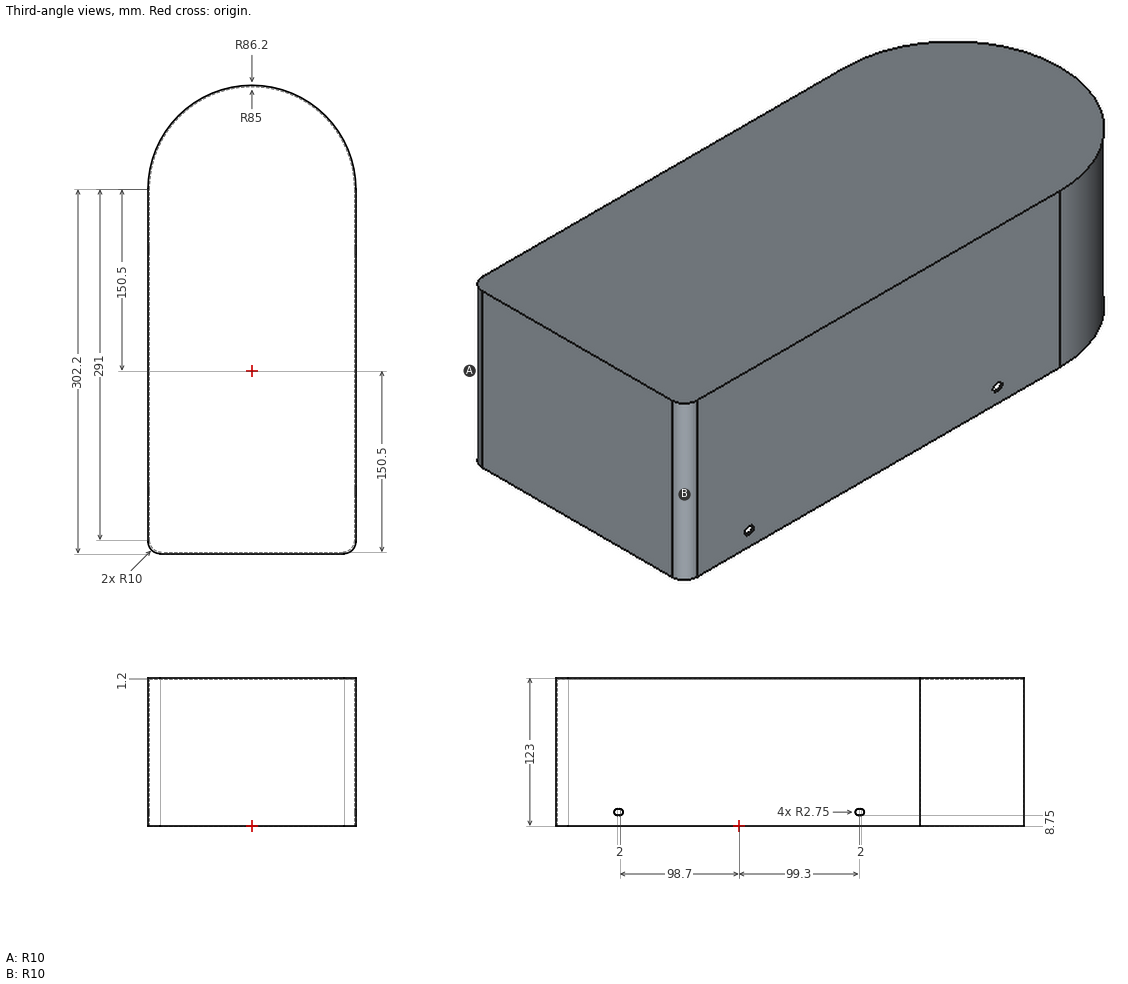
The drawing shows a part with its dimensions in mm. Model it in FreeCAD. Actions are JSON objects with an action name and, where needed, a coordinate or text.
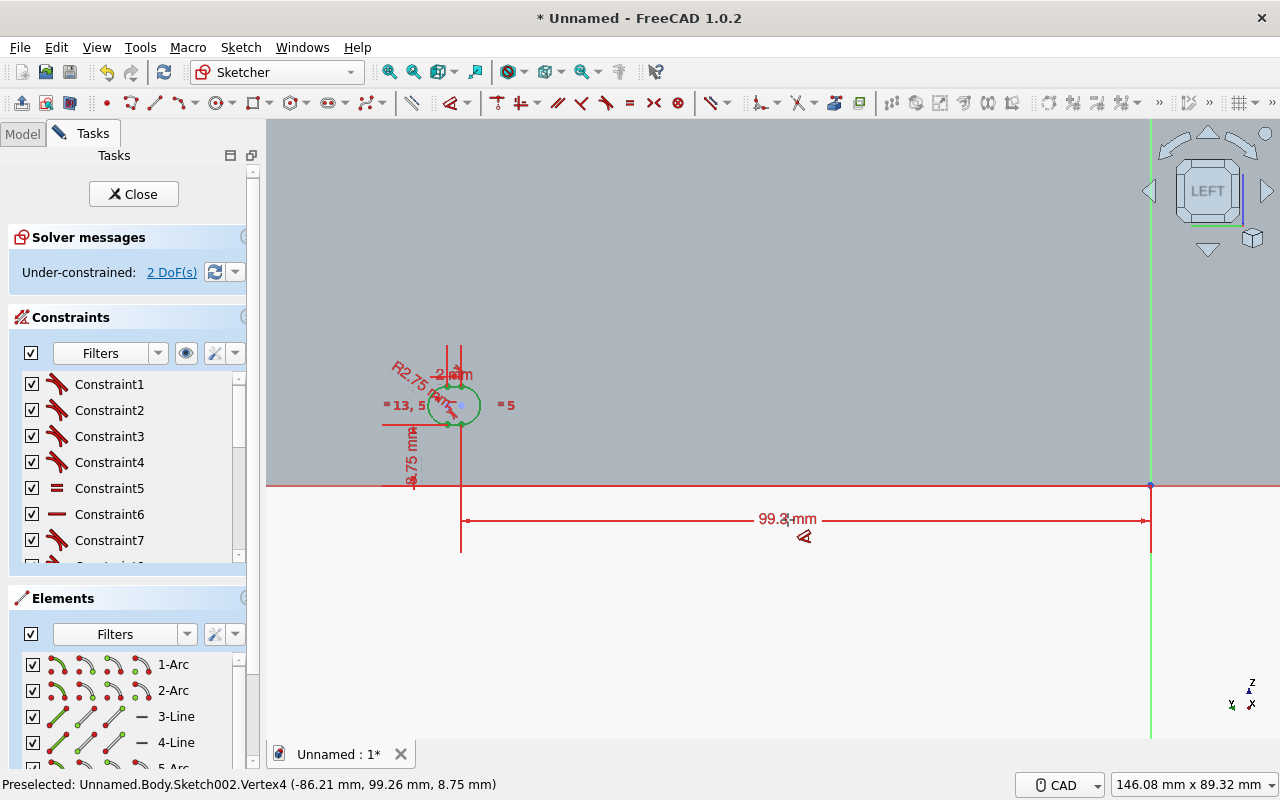
{"action": "scroll", "coordinate": [446, 425], "scroll_direction": "down", "scroll_amount": 5}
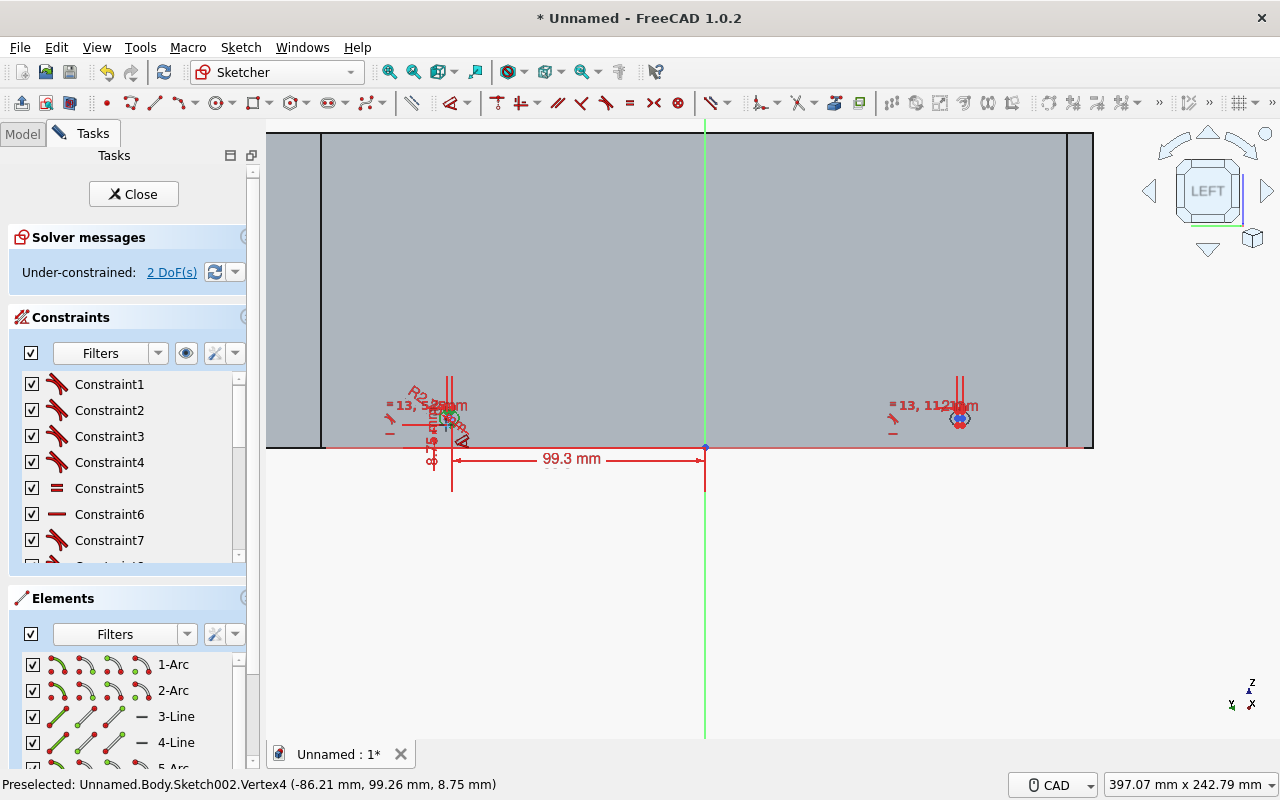
{"action": "scroll", "coordinate": [957, 412], "scroll_direction": "up", "scroll_amount": 5}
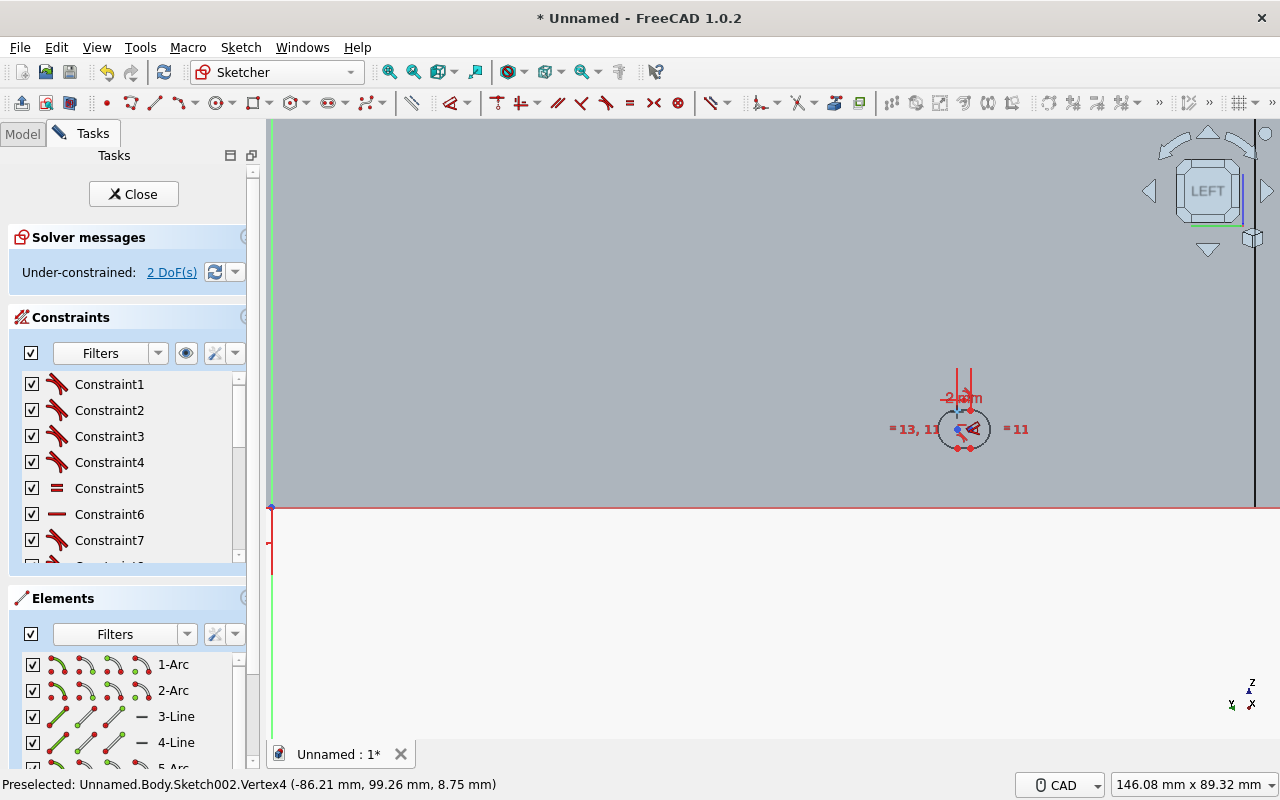
{"action": "left_click", "coordinate": [957, 410]}
{"action": "left_click", "coordinate": [626, 542]}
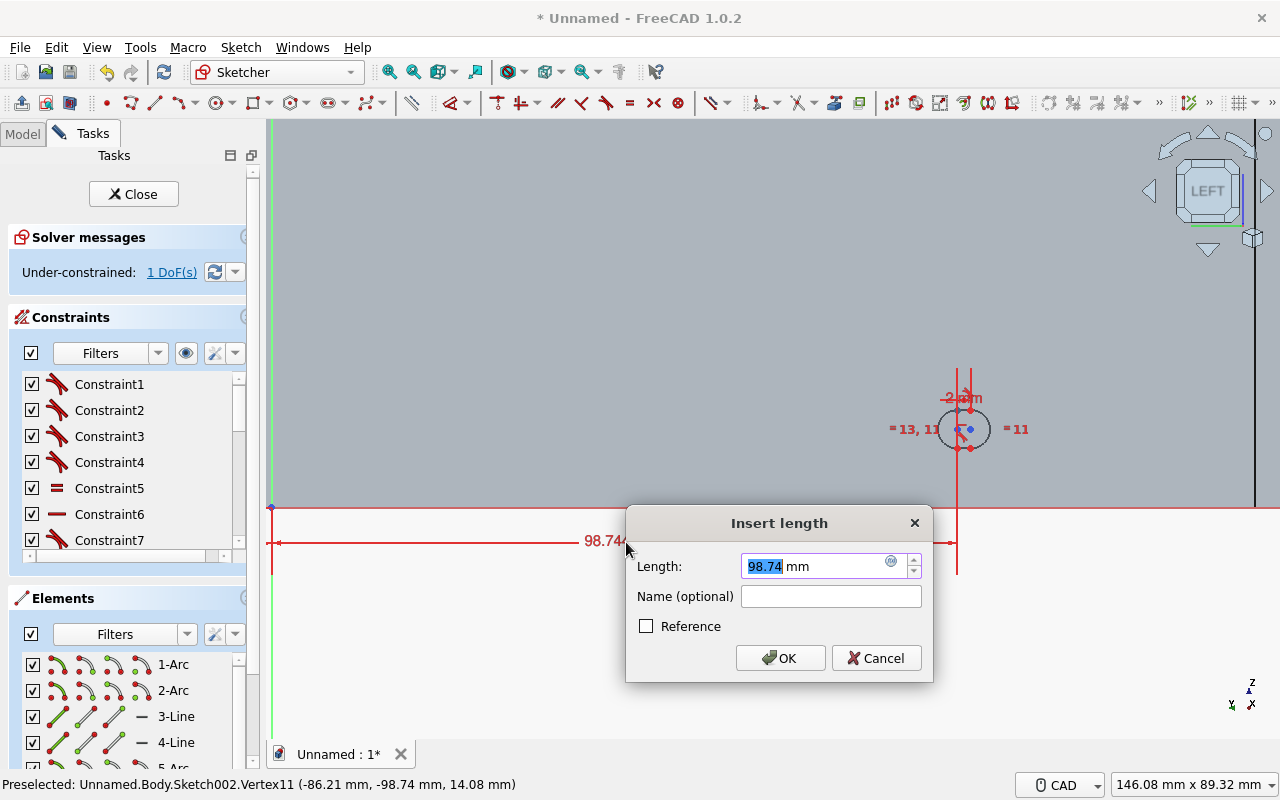
{"action": "type", "text": "98.7"}
{"action": "key", "text": "Return"}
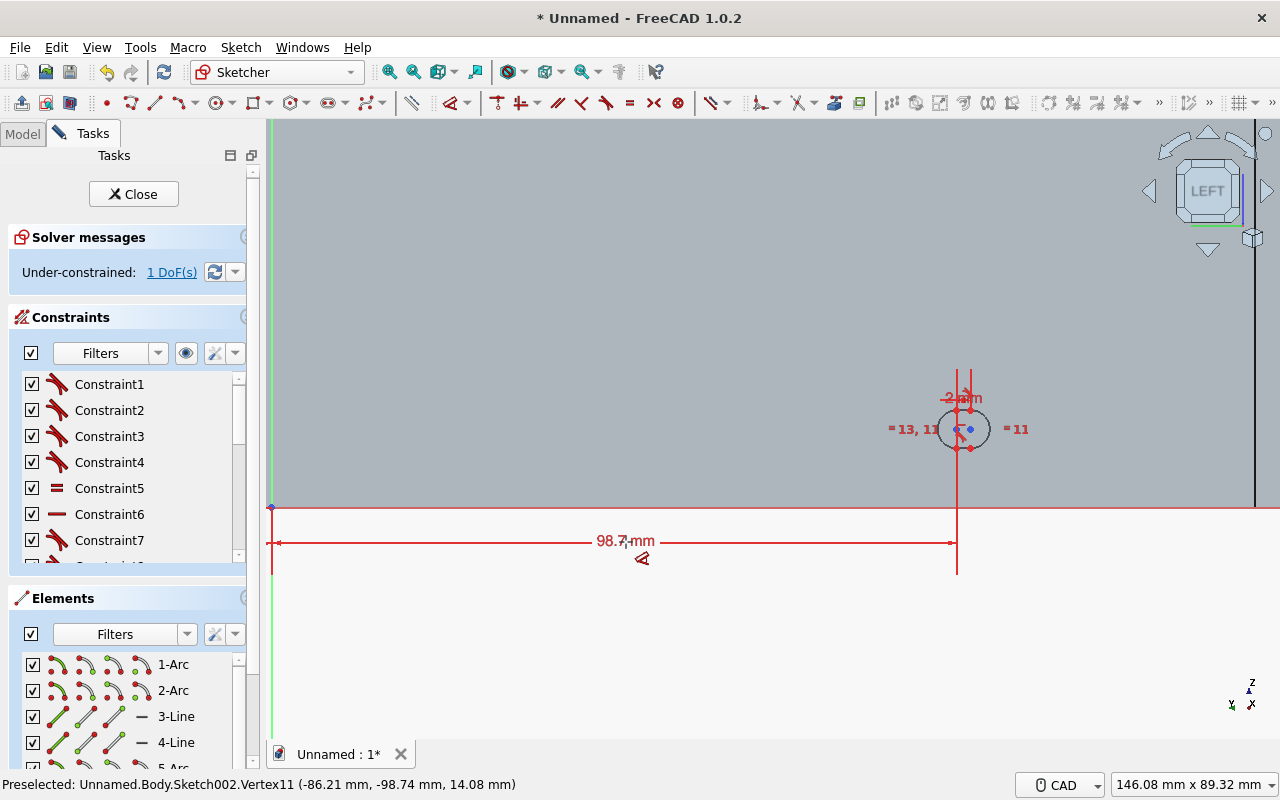
{"action": "left_click", "coordinate": [957, 448]}
{"action": "left_click", "coordinate": [991, 478]}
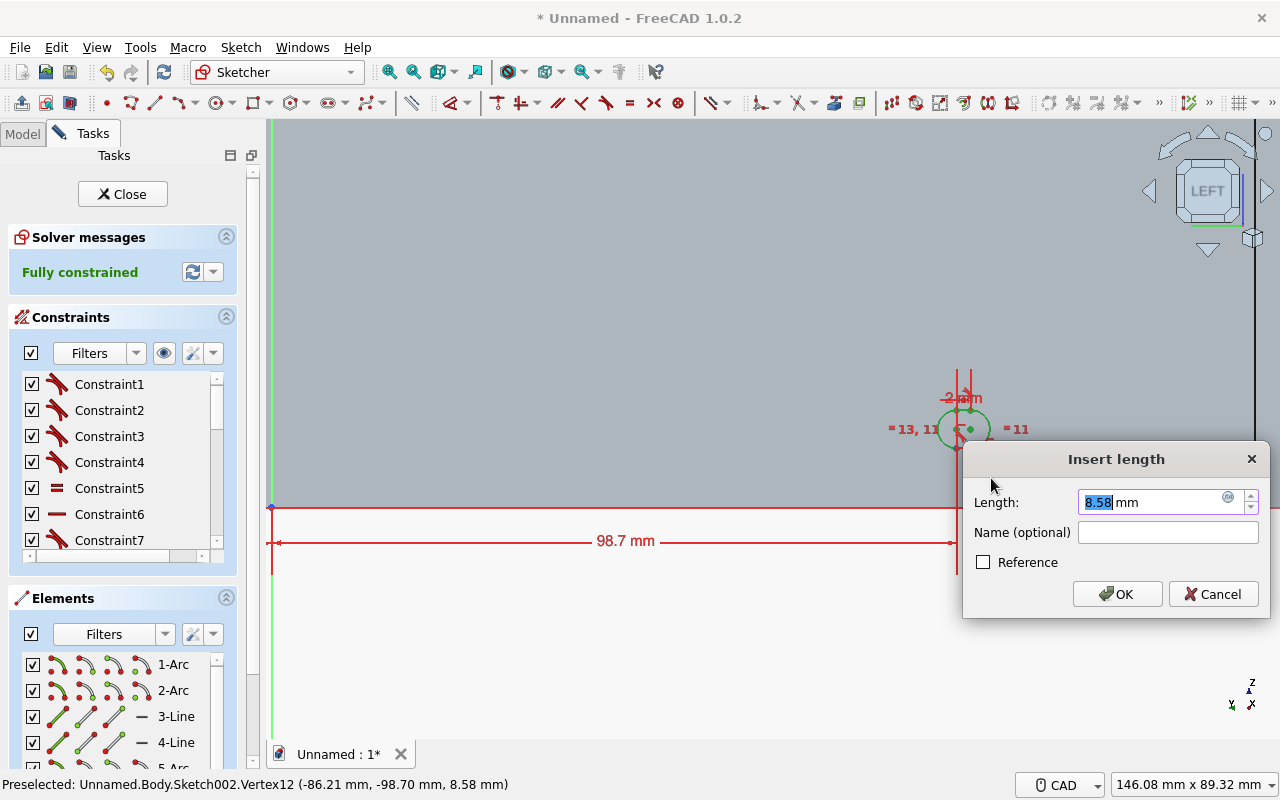
{"action": "type", "text": "8.75"}
{"action": "key", "text": "Return"}
{"action": "key", "text": "Escape"}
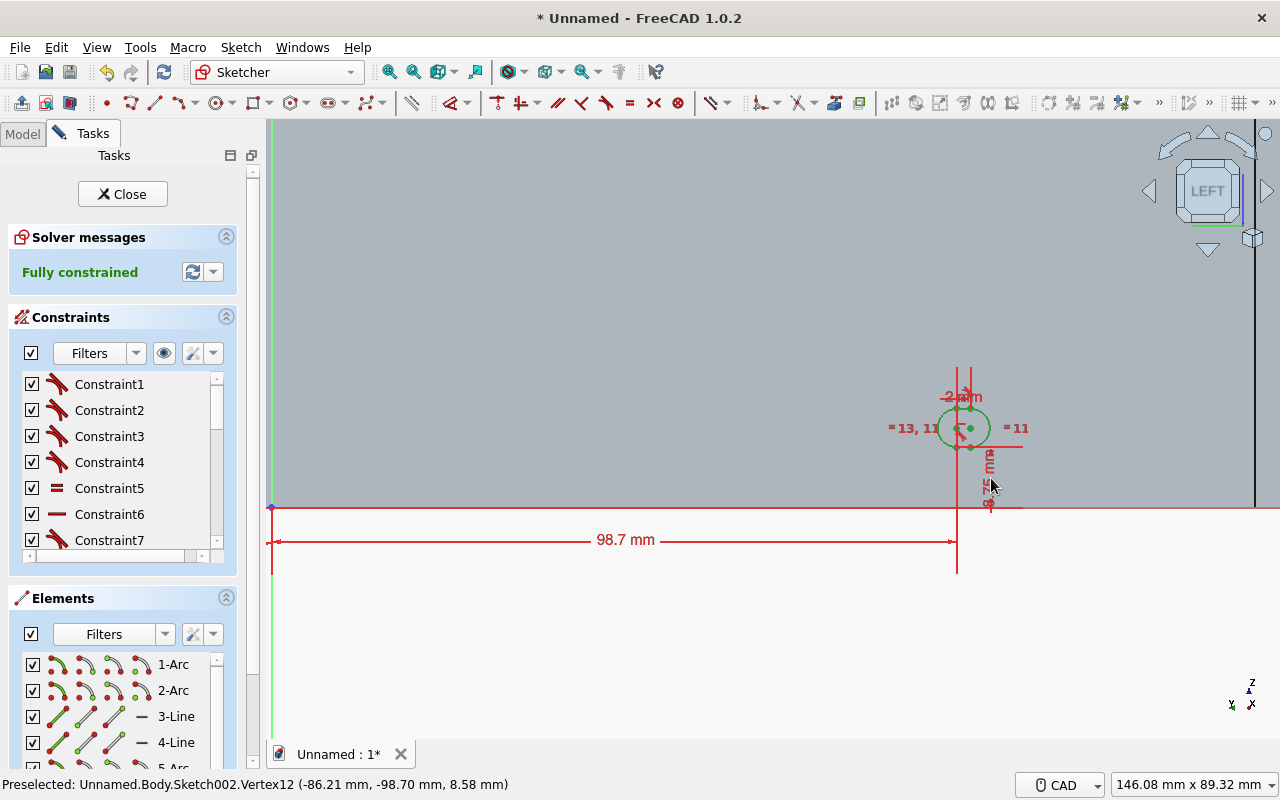
{"action": "left_click", "coordinate": [123, 194]}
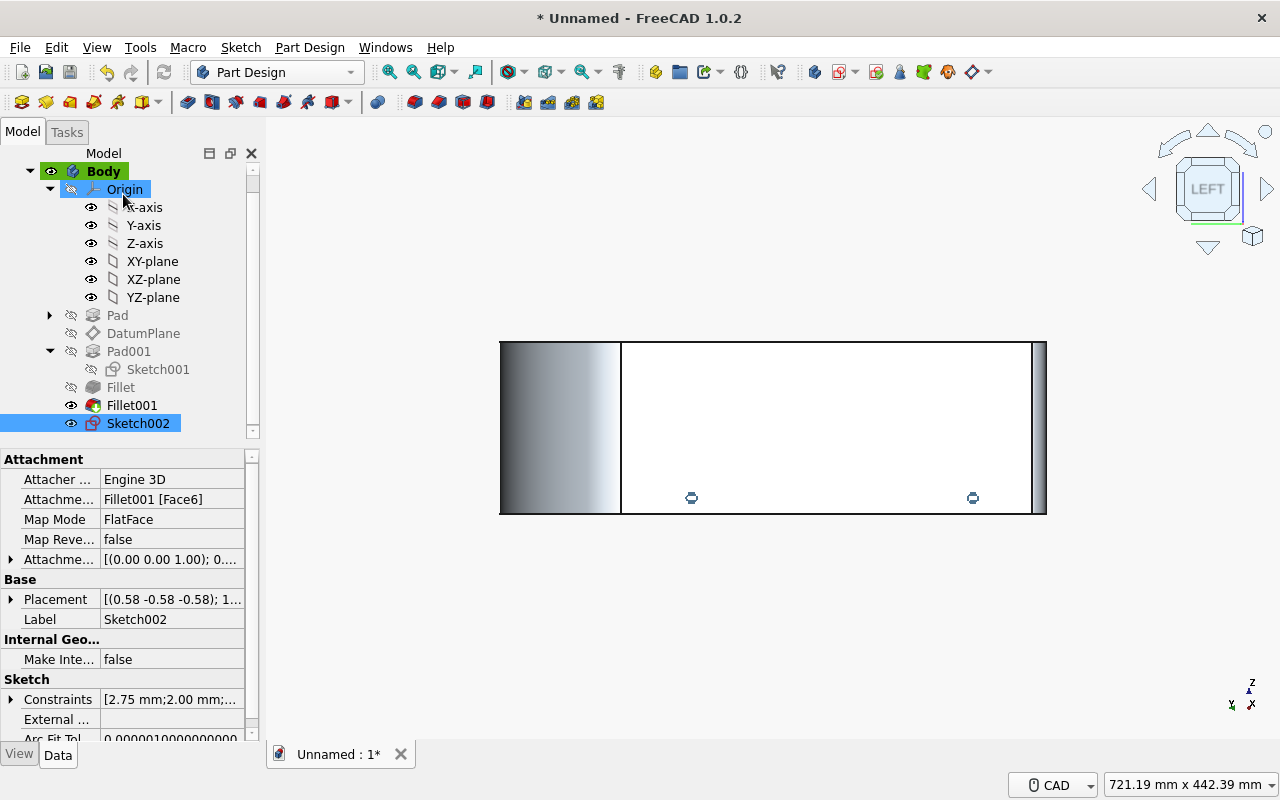
{"action": "left_click", "coordinate": [188, 102]}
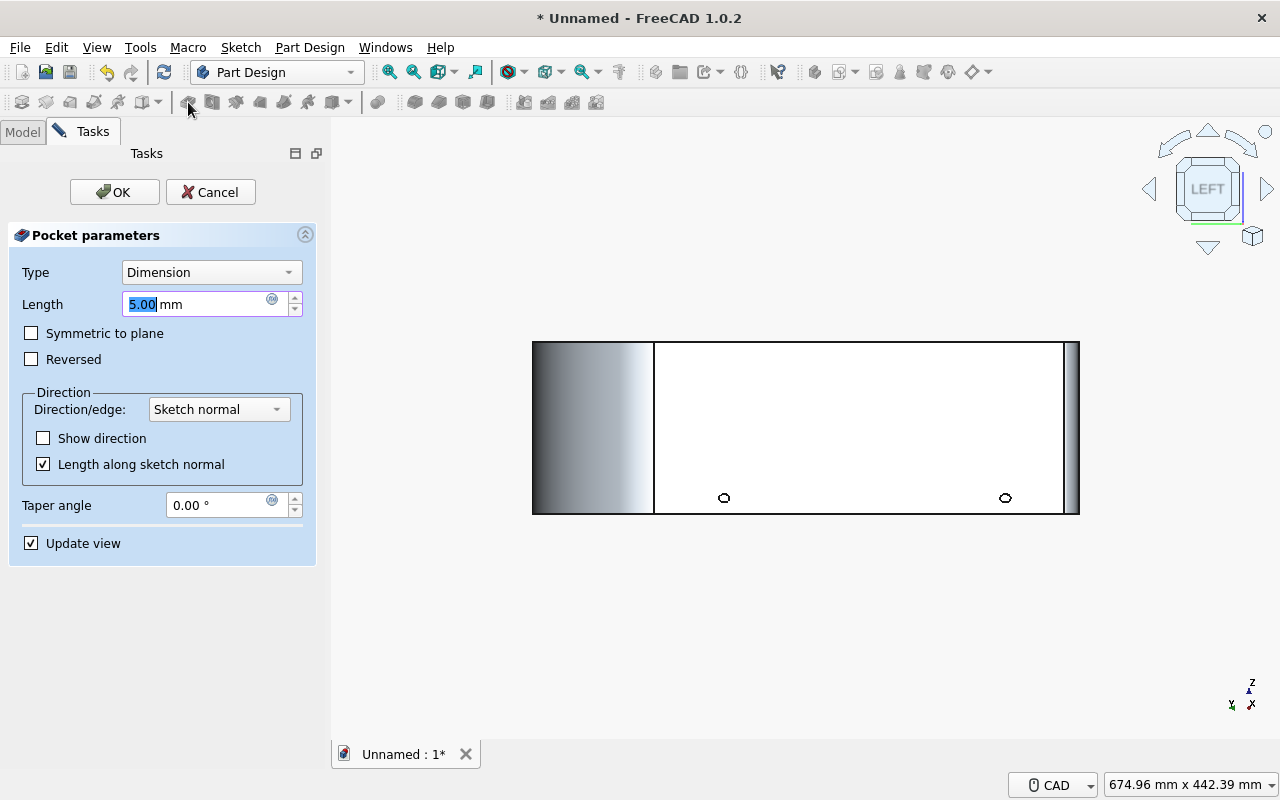
{"action": "left_click", "coordinate": [212, 272]}